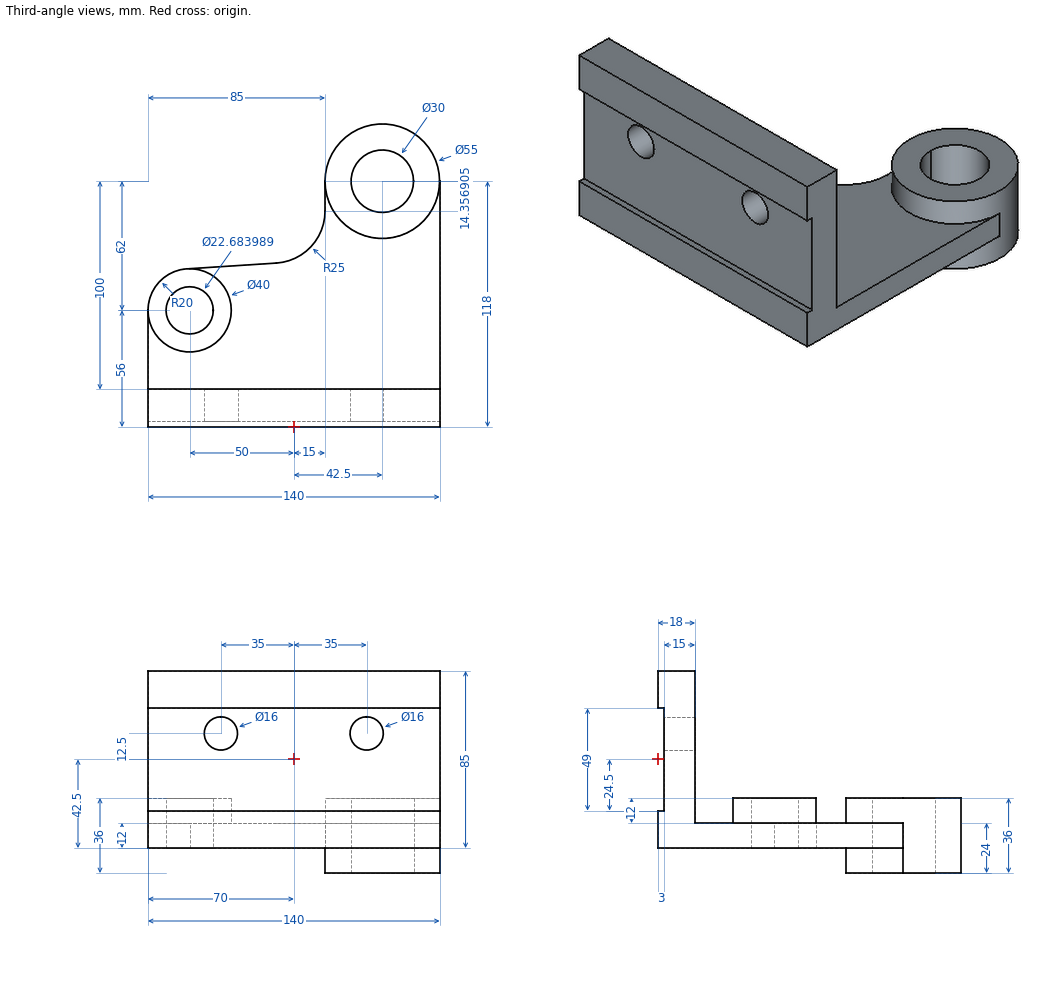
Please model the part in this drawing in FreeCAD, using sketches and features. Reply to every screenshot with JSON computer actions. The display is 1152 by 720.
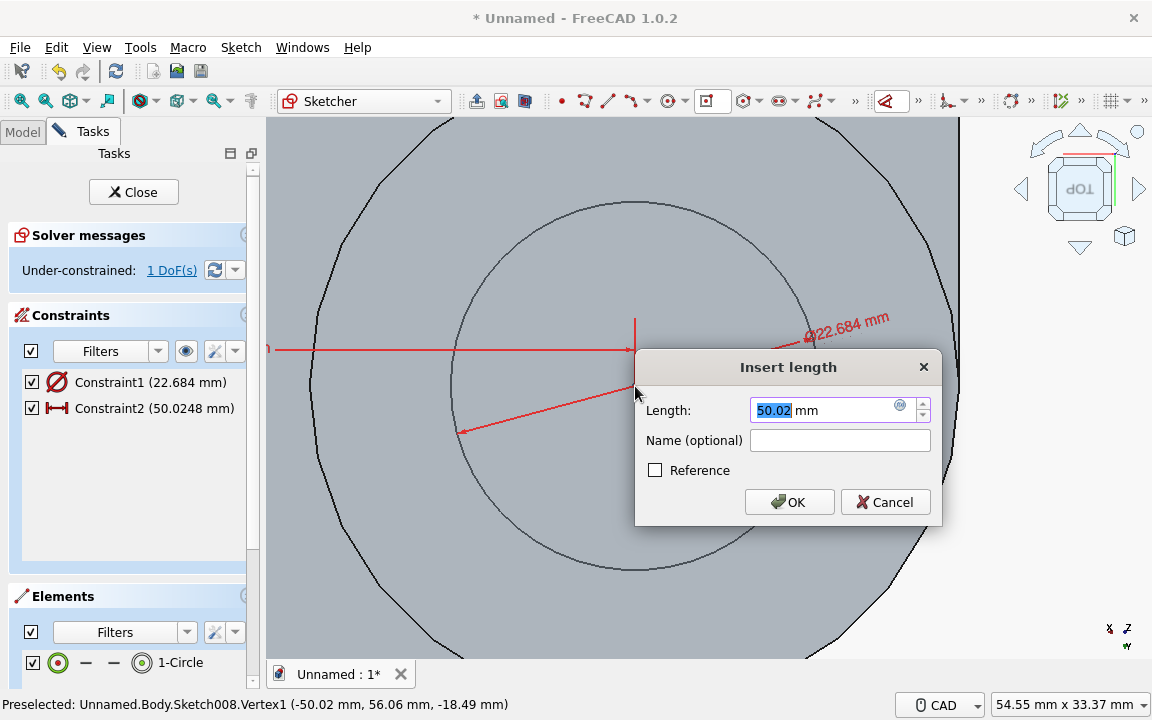
{"action": "type", "text": "50"}
{"action": "key", "text": "Return"}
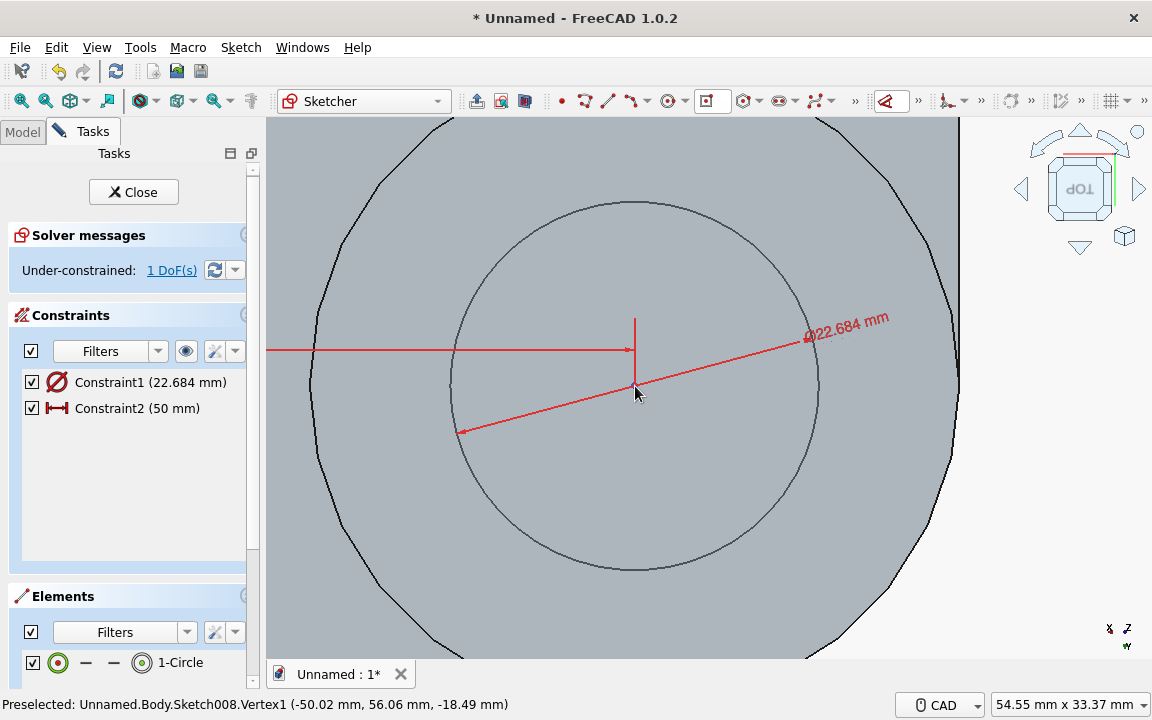
{"action": "left_click", "coordinate": [635, 386]}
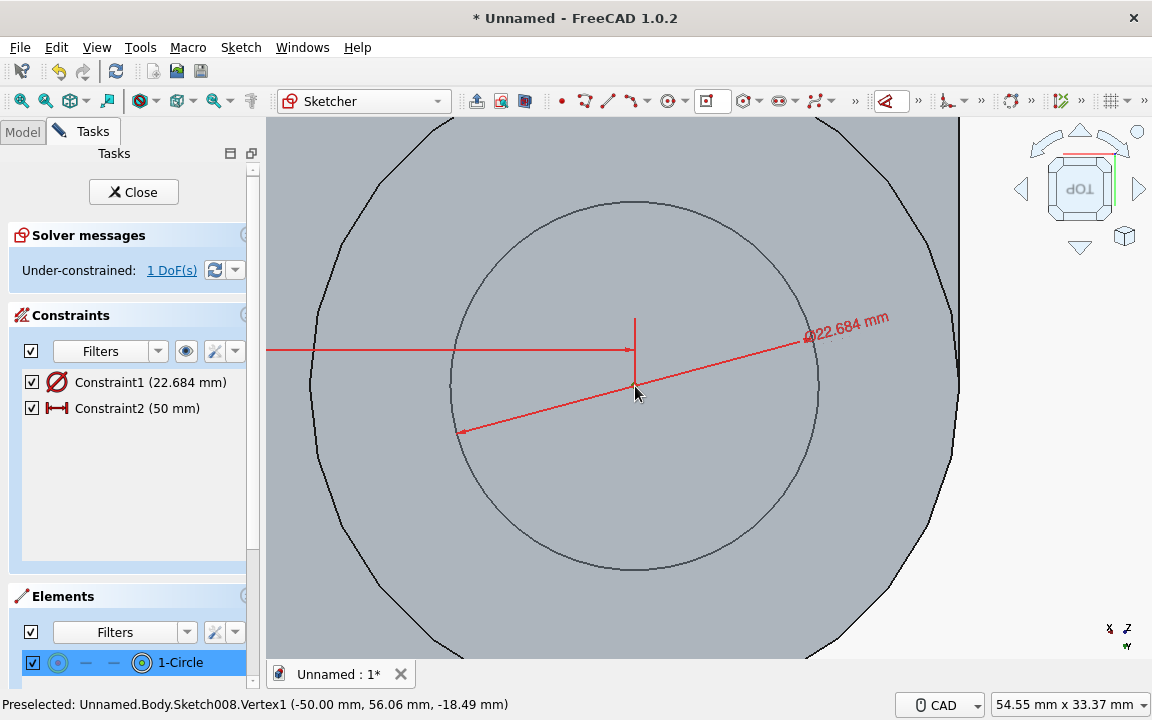
{"action": "key", "text": "i"}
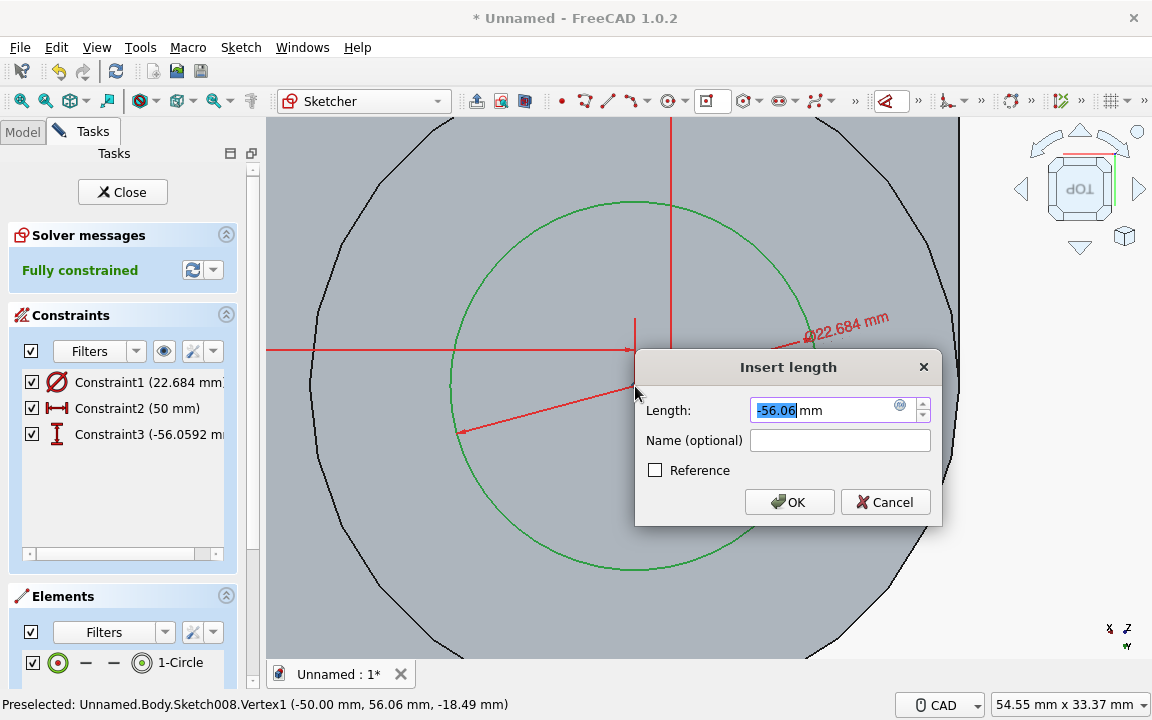
{"action": "type", "text": "-56"}
{"action": "key", "text": "Return"}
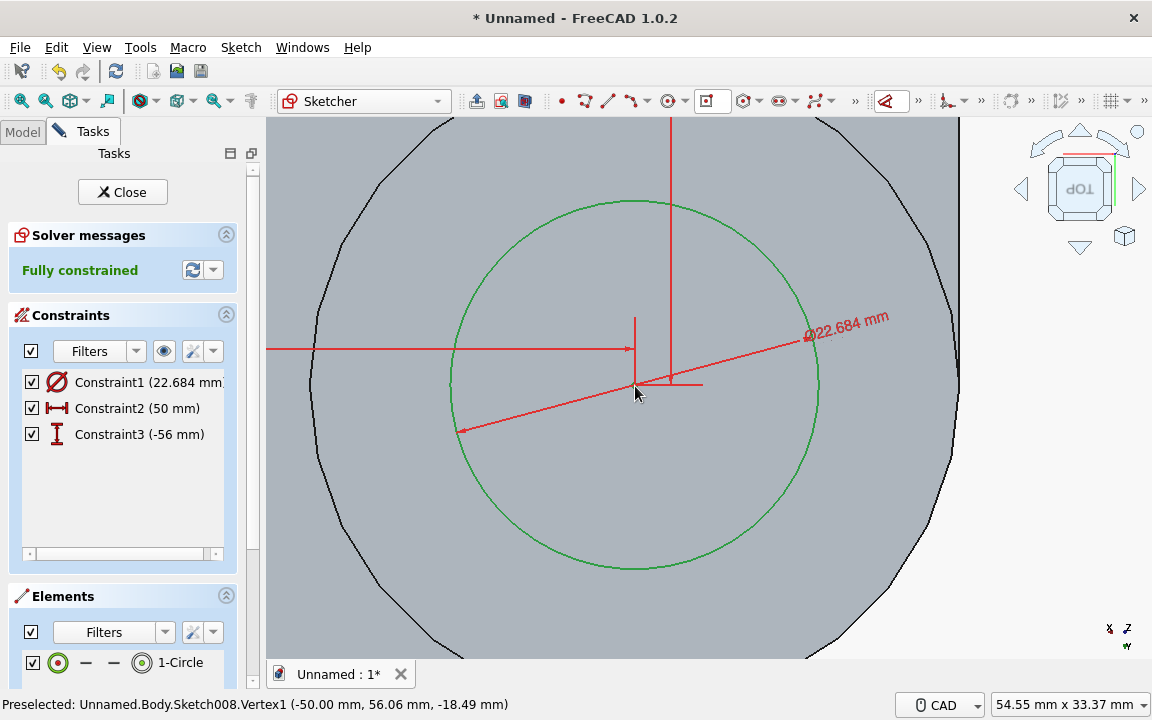
{"action": "left_click", "coordinate": [123, 192]}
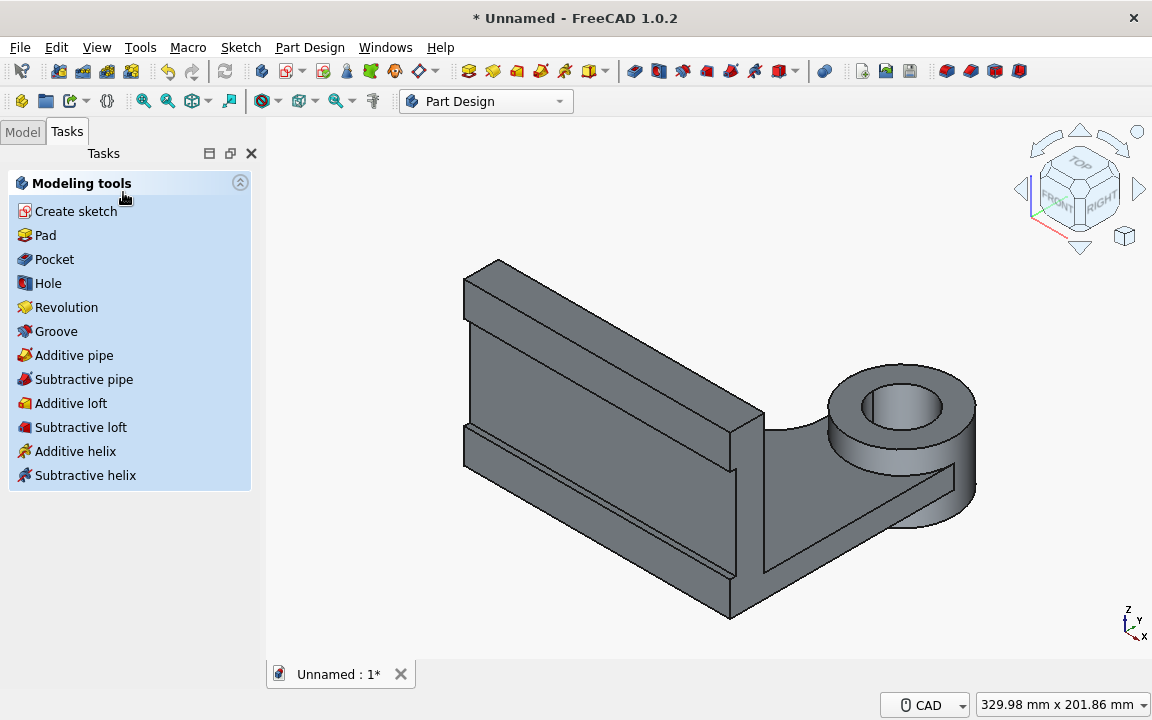
{"action": "left_click", "coordinate": [636, 72]}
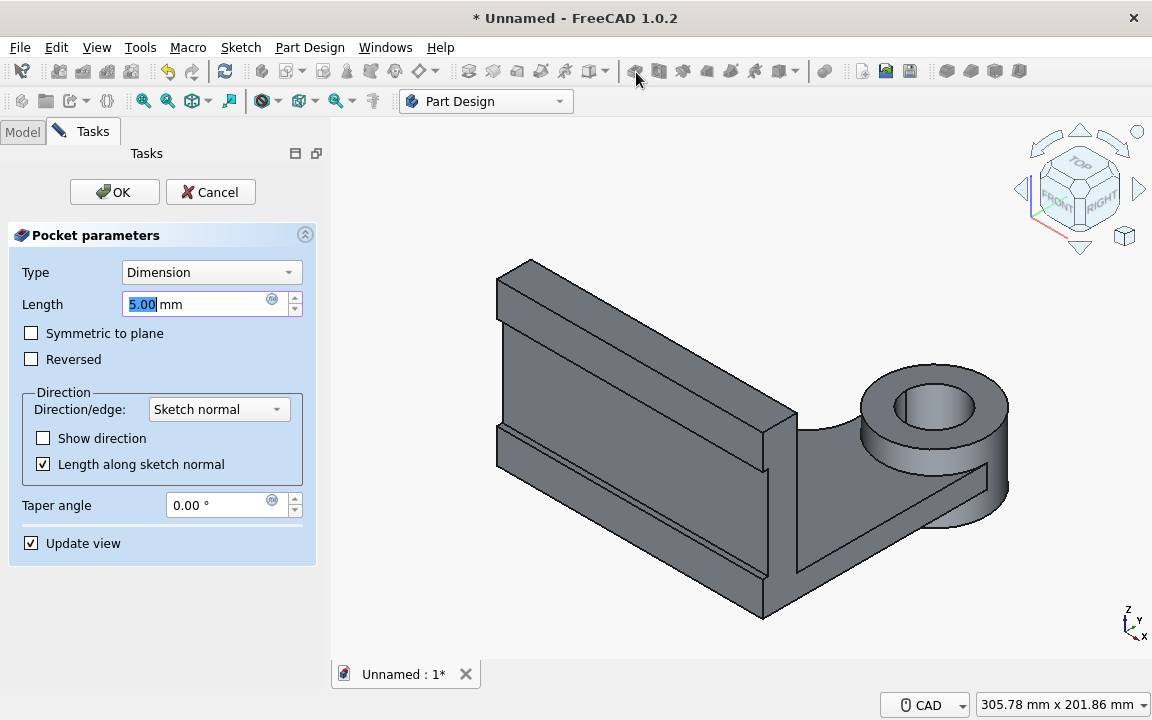
{"action": "type", "text": "36"}
{"action": "key", "text": "Tab"}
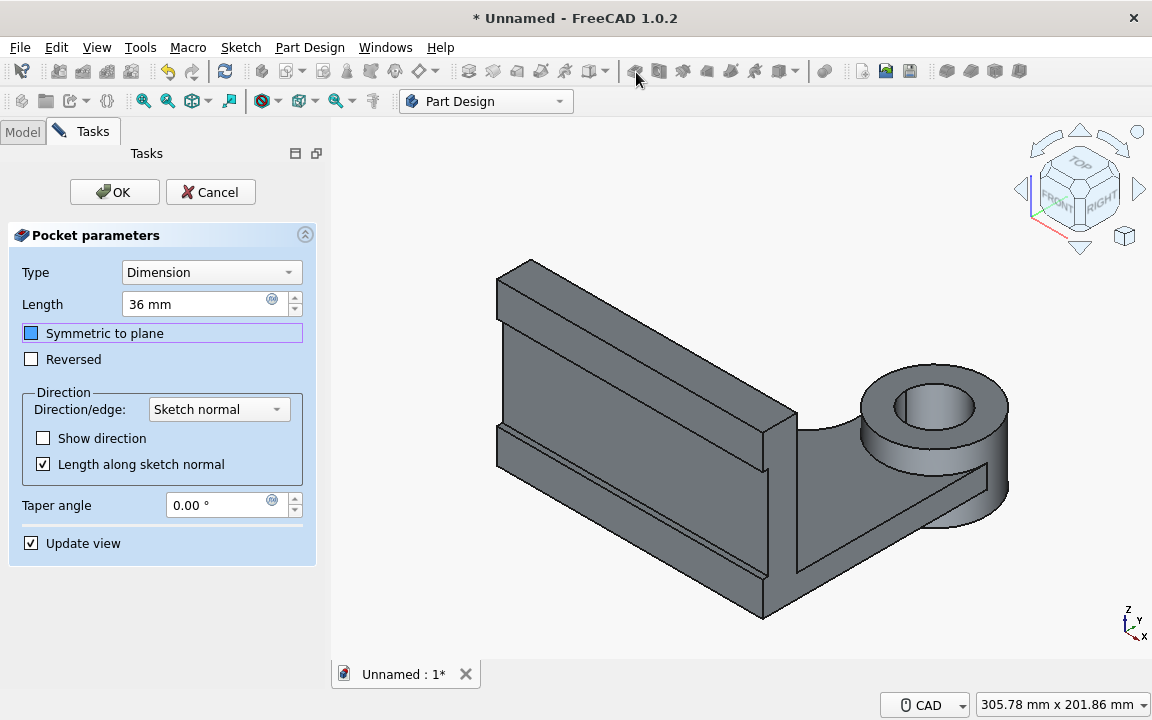
{"action": "left_click", "coordinate": [115, 192]}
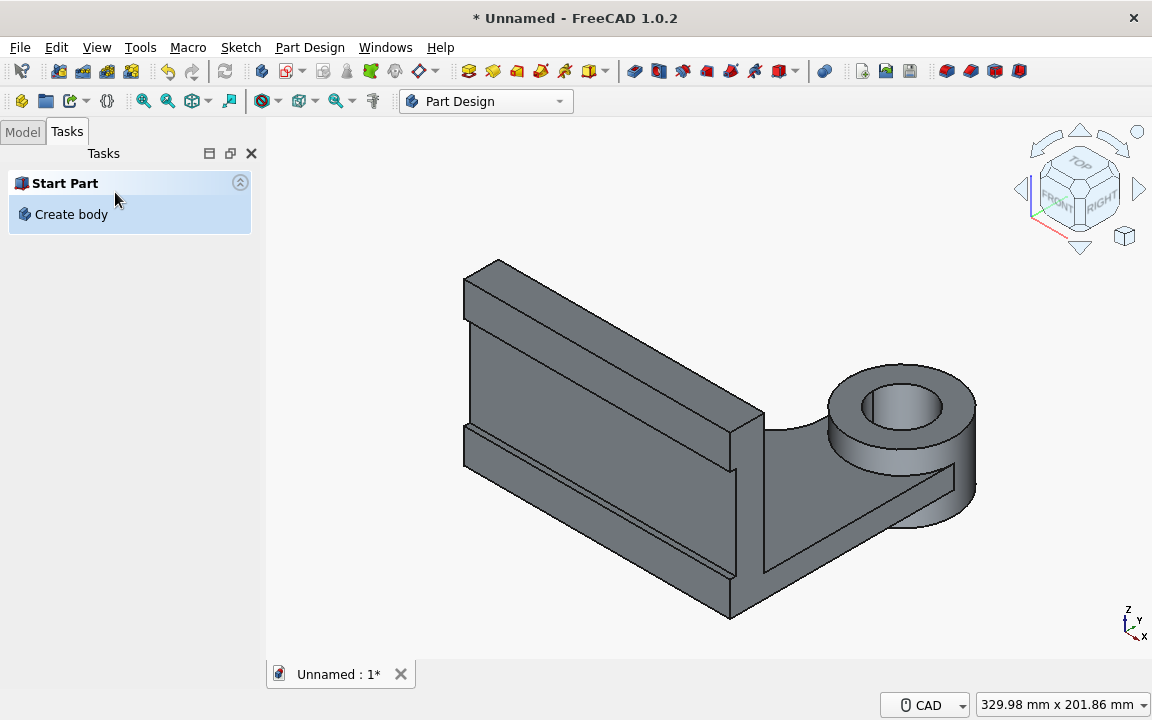
{"action": "key", "text": "4"}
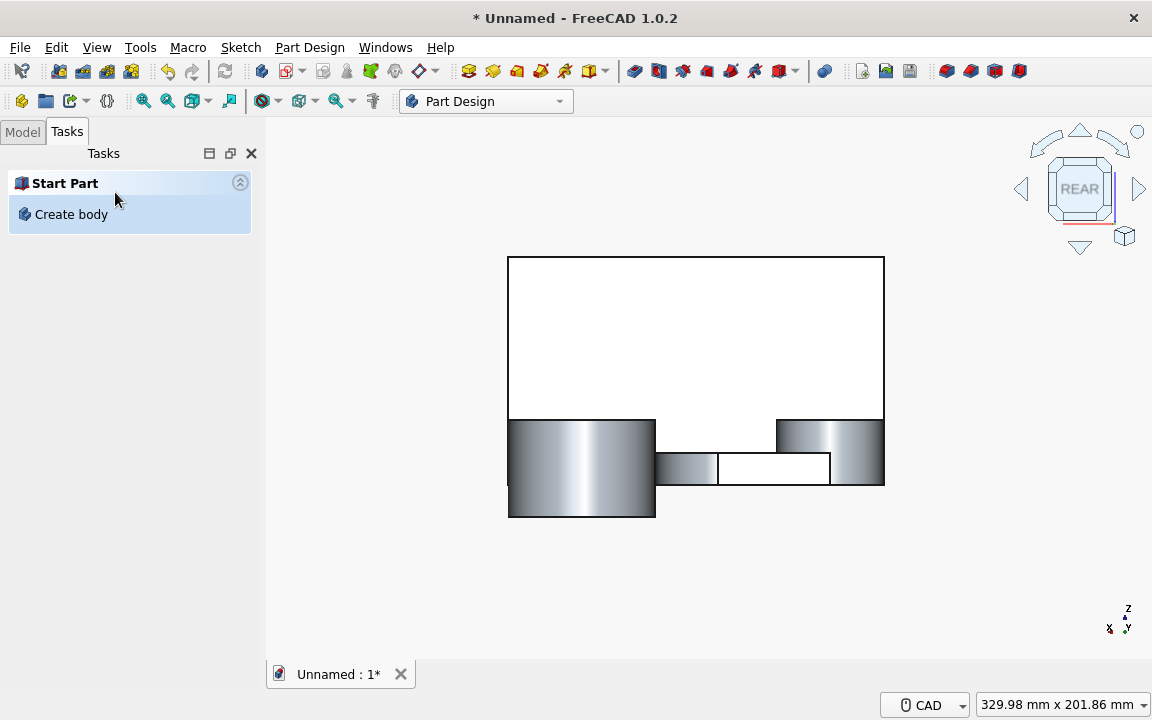
{"action": "left_click", "coordinate": [642, 354]}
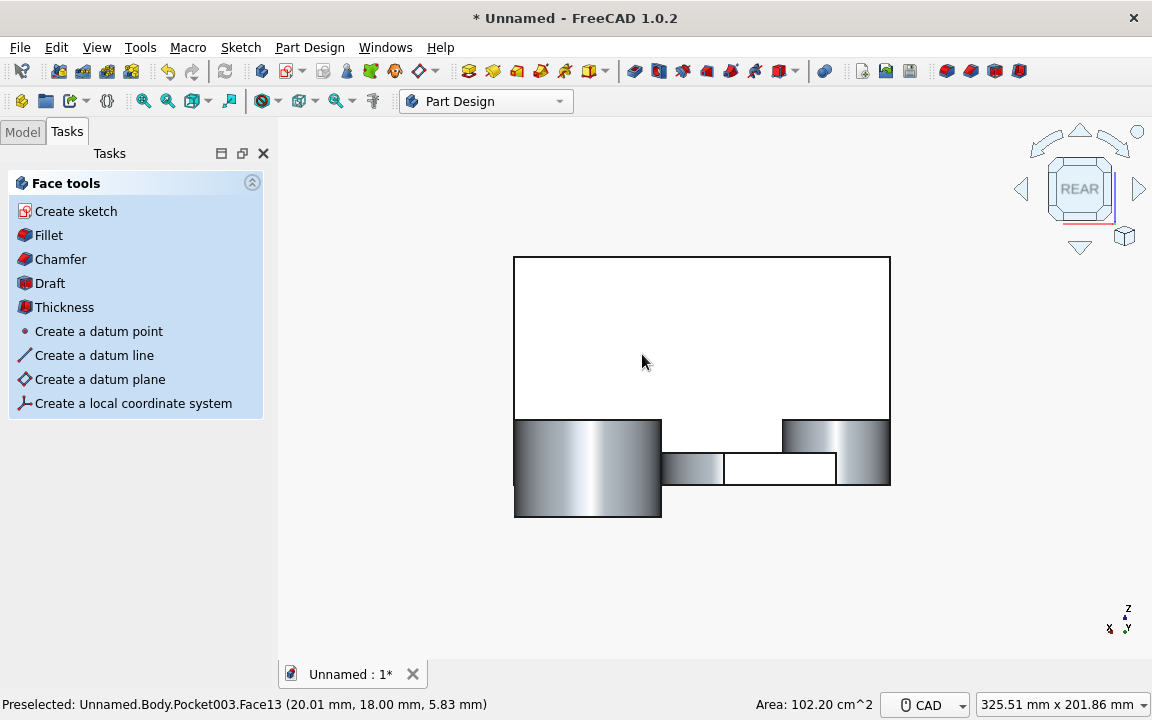
{"action": "left_click", "coordinate": [286, 72]}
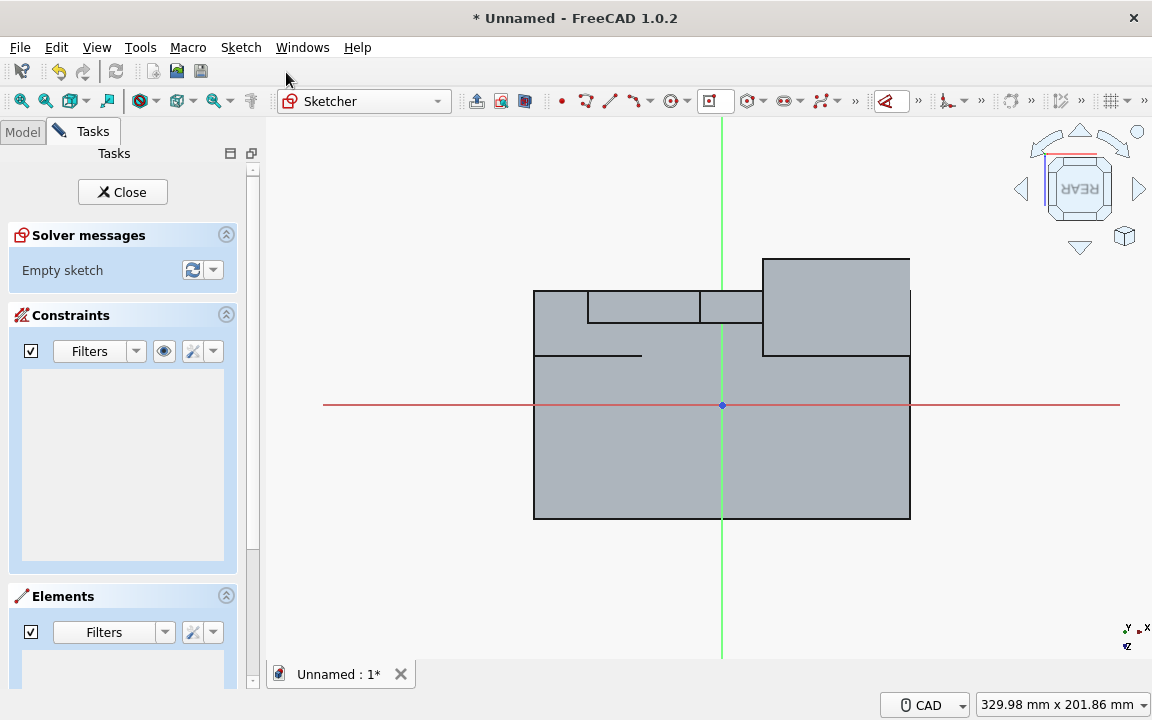
{"action": "scroll", "coordinate": [626, 447], "scroll_direction": "up", "scroll_amount": 10}